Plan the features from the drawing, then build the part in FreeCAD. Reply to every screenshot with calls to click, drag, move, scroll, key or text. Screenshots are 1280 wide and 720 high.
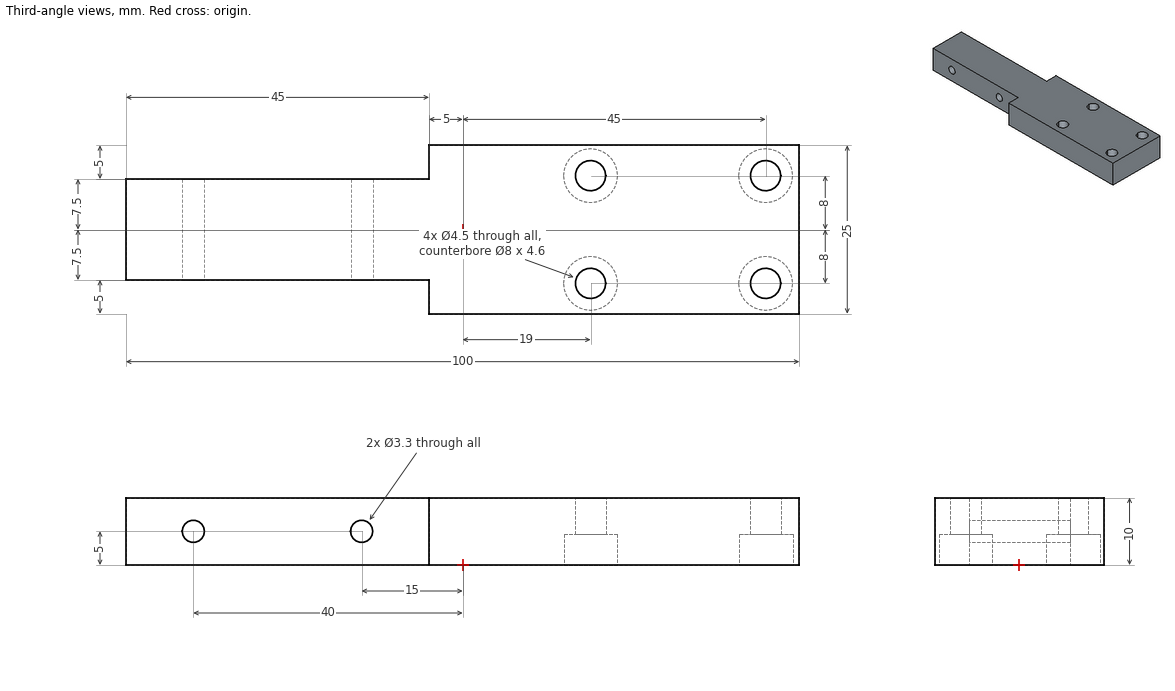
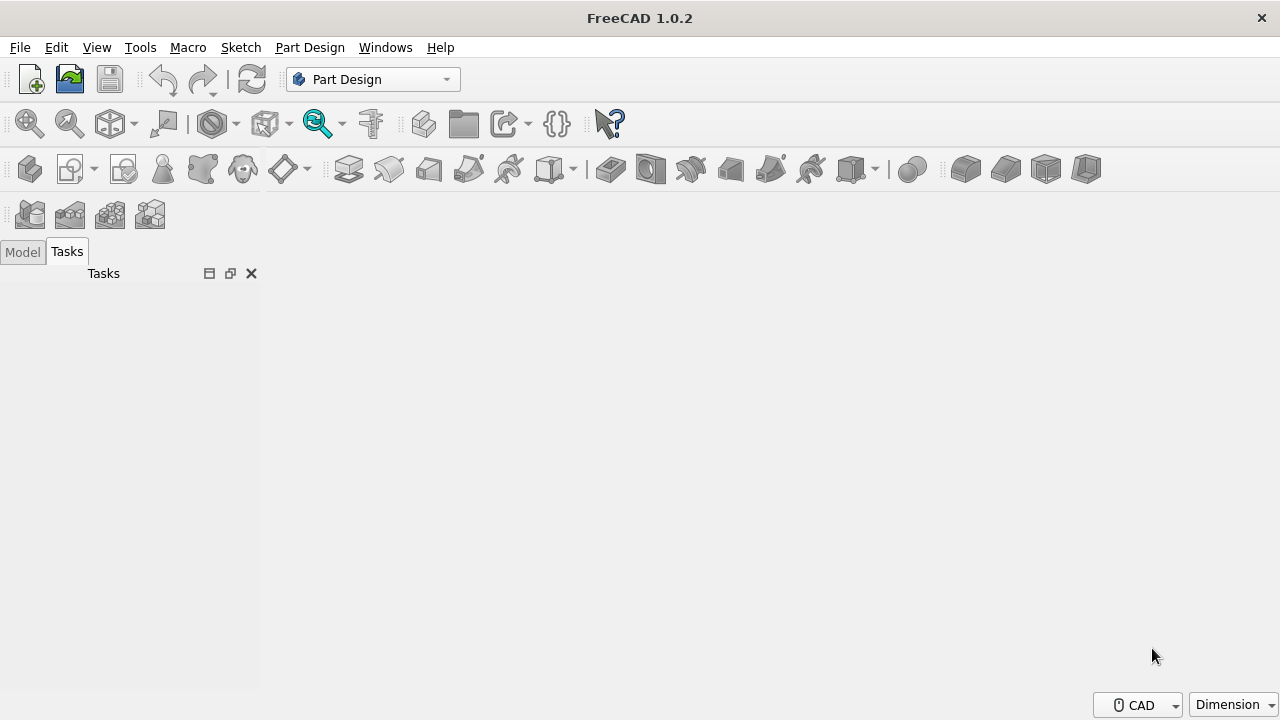
click(548, 80)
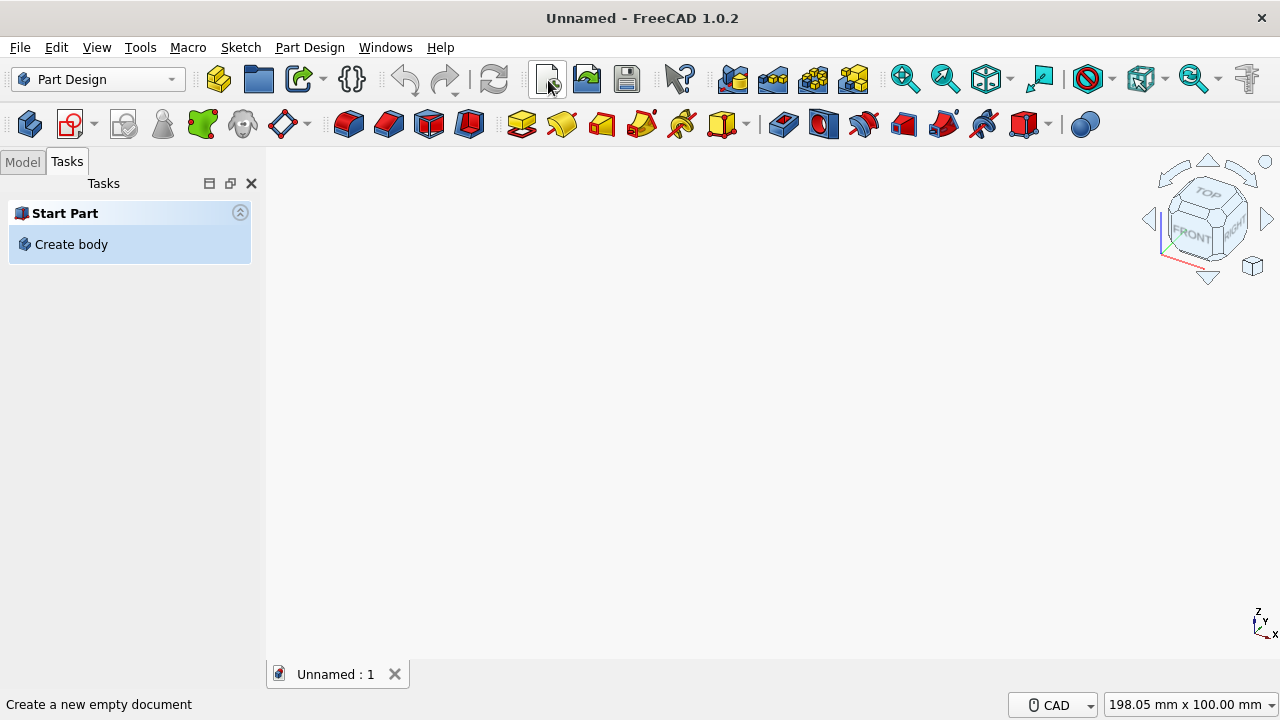
click(70, 124)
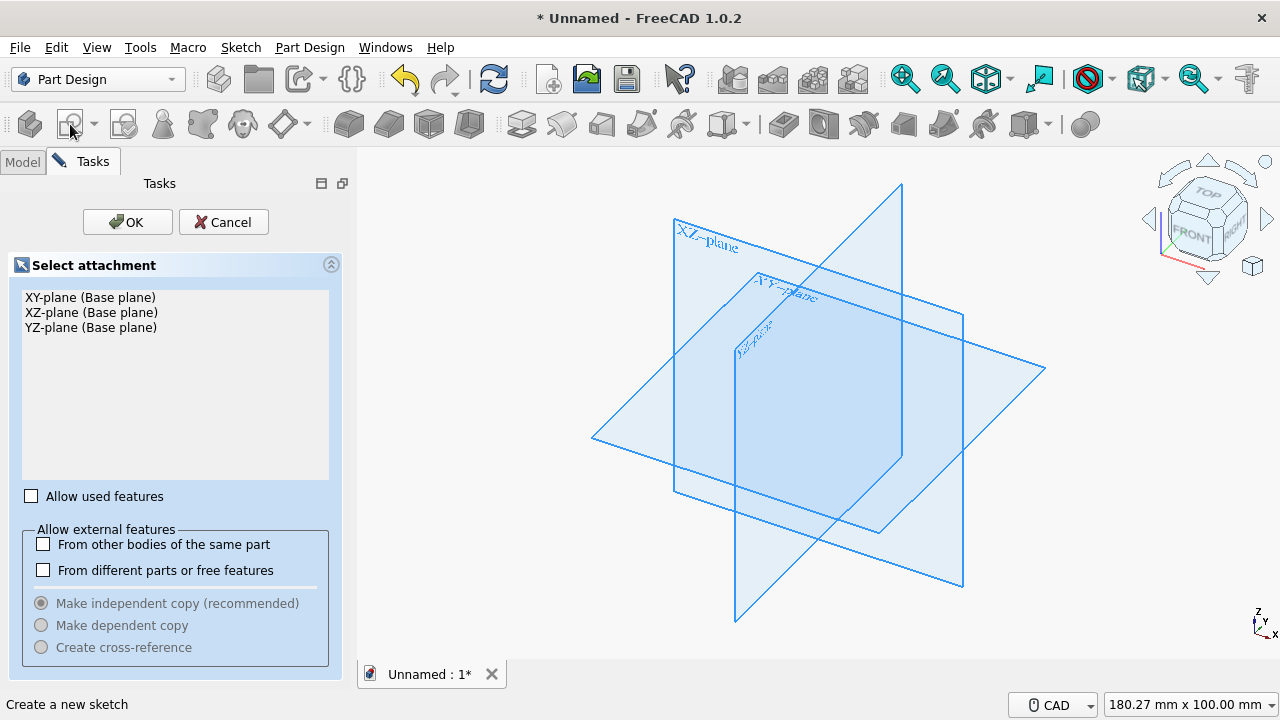
click(82, 298)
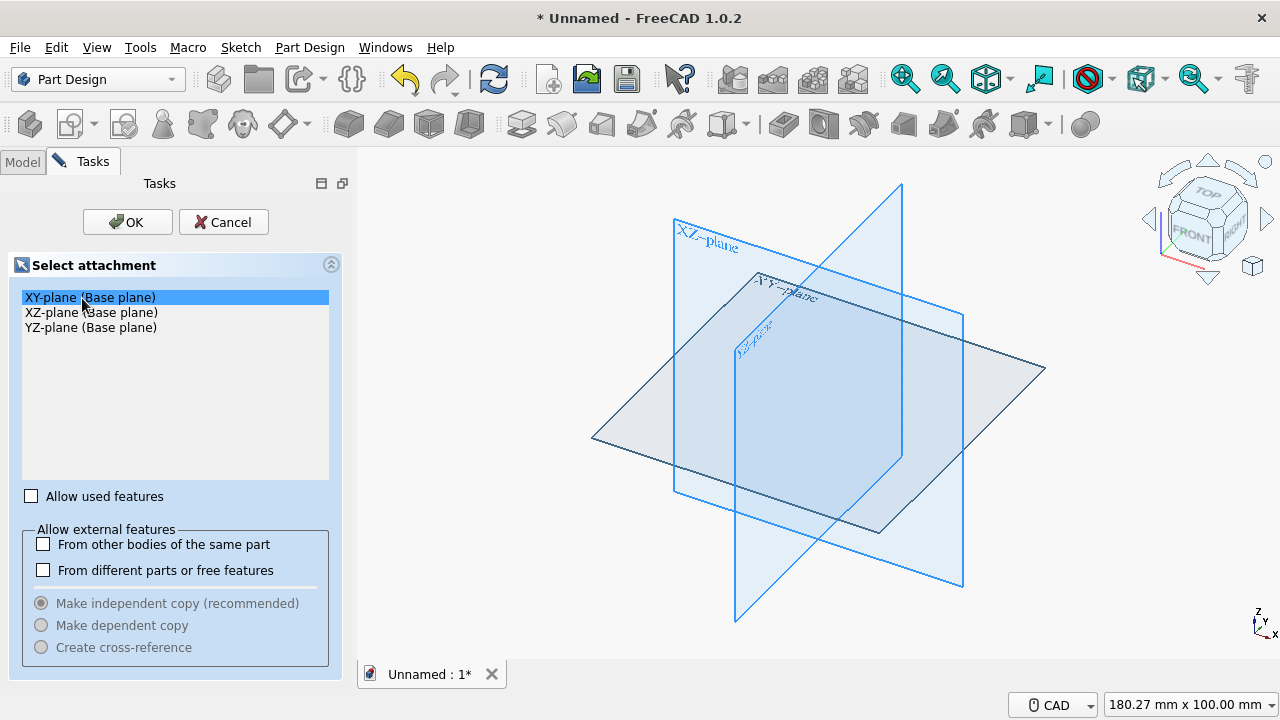
click(128, 222)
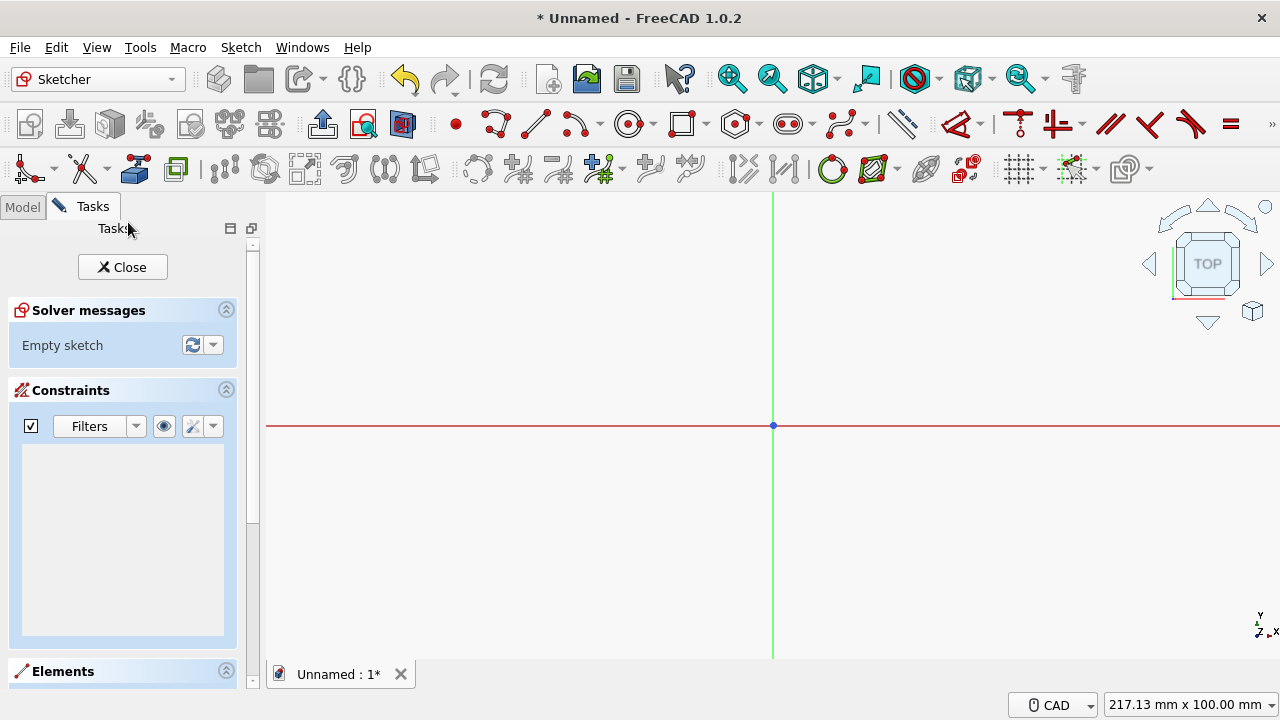
click(708, 124)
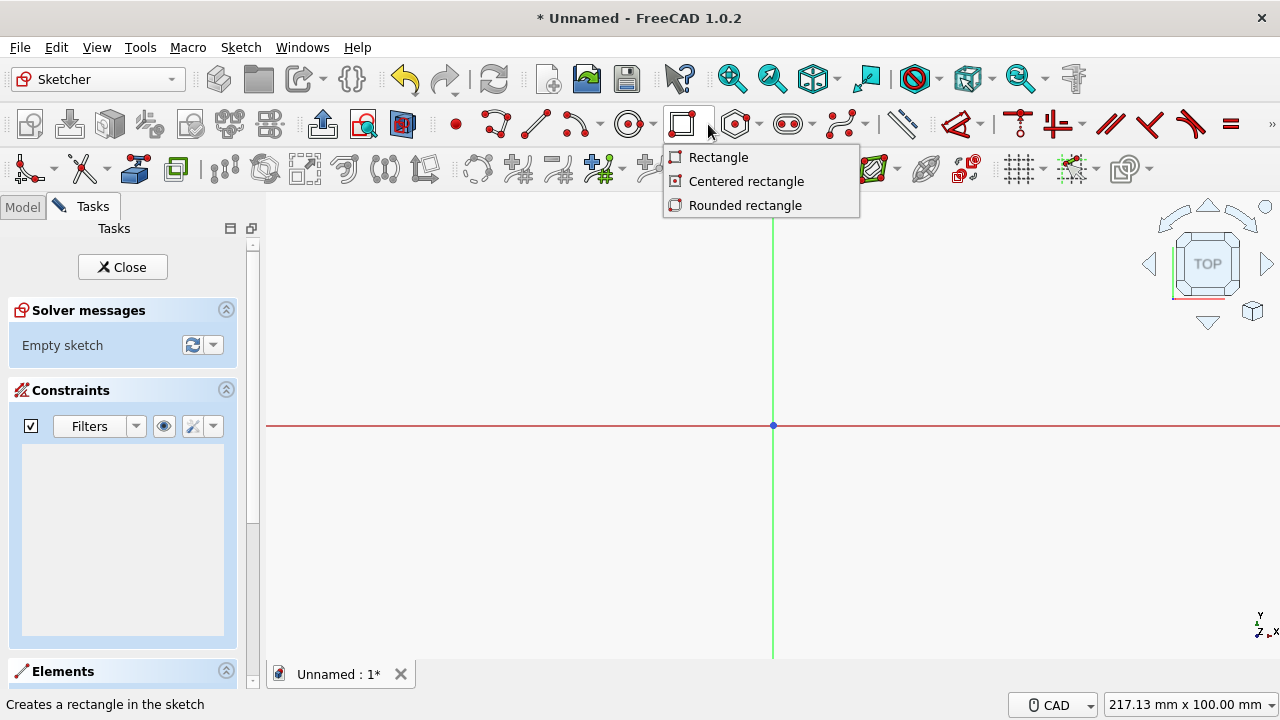
click(762, 181)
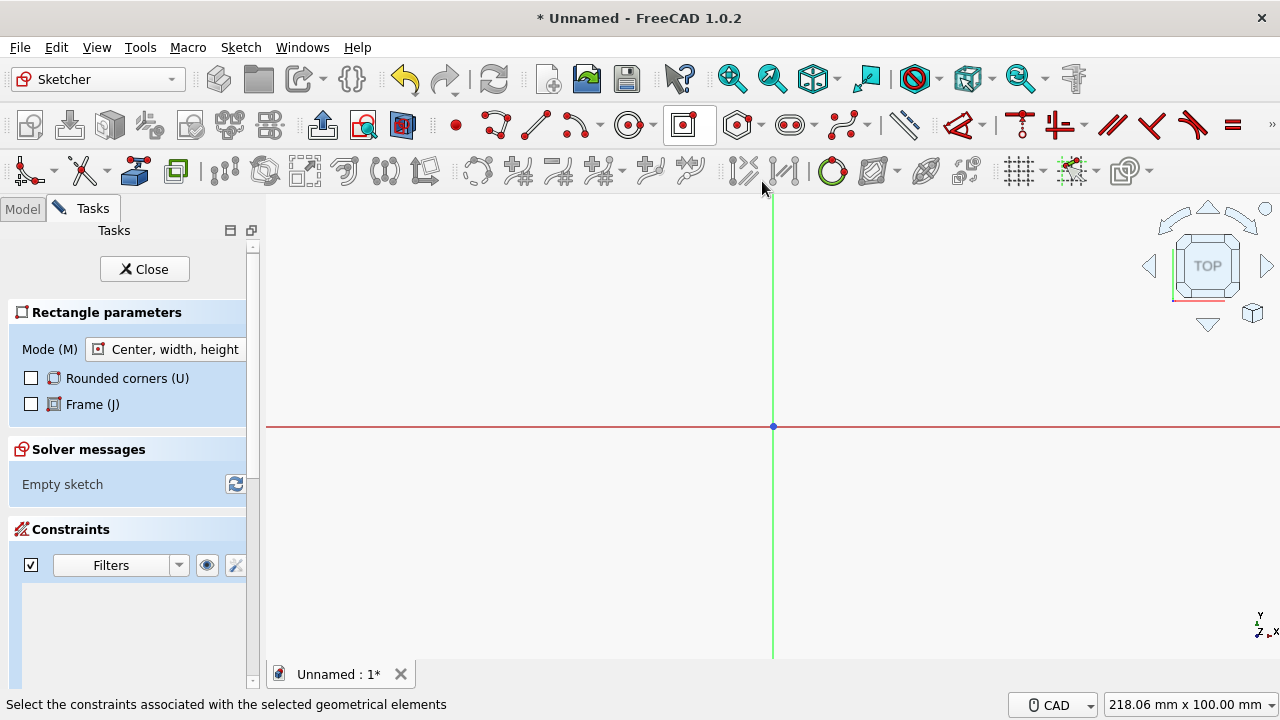
click(773, 426)
click(1006, 368)
key(Escape)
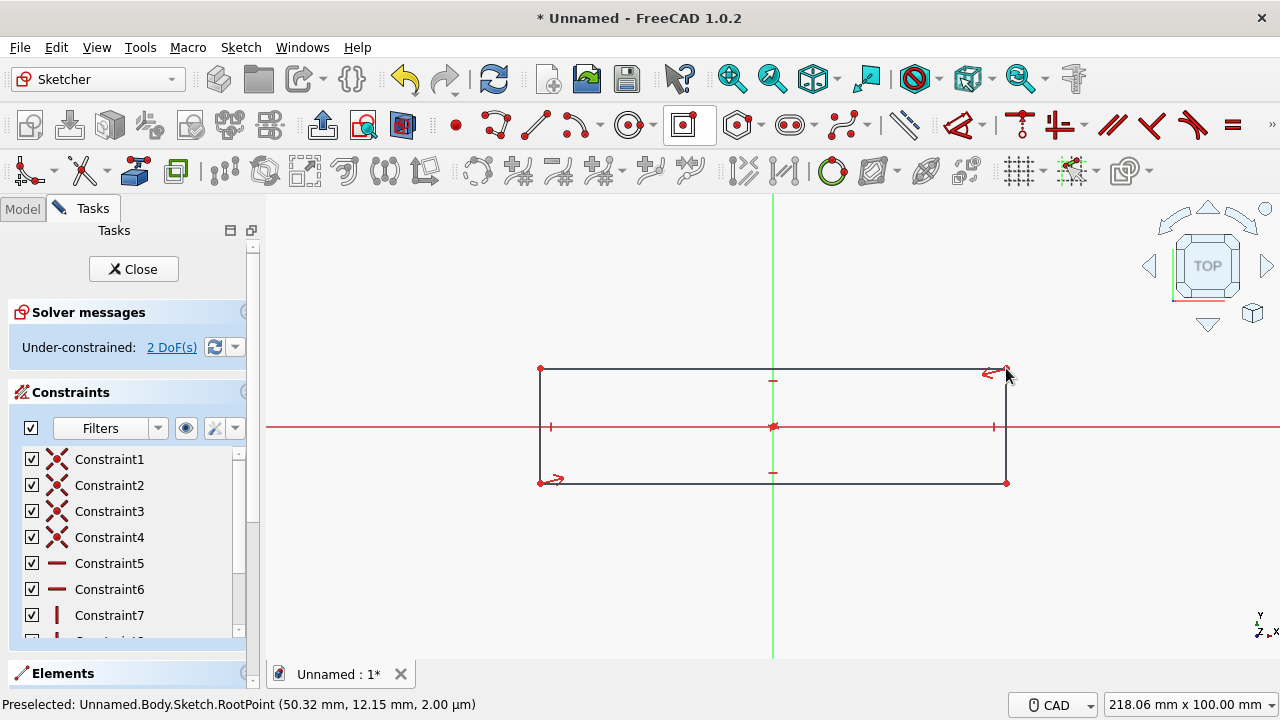
click(958, 126)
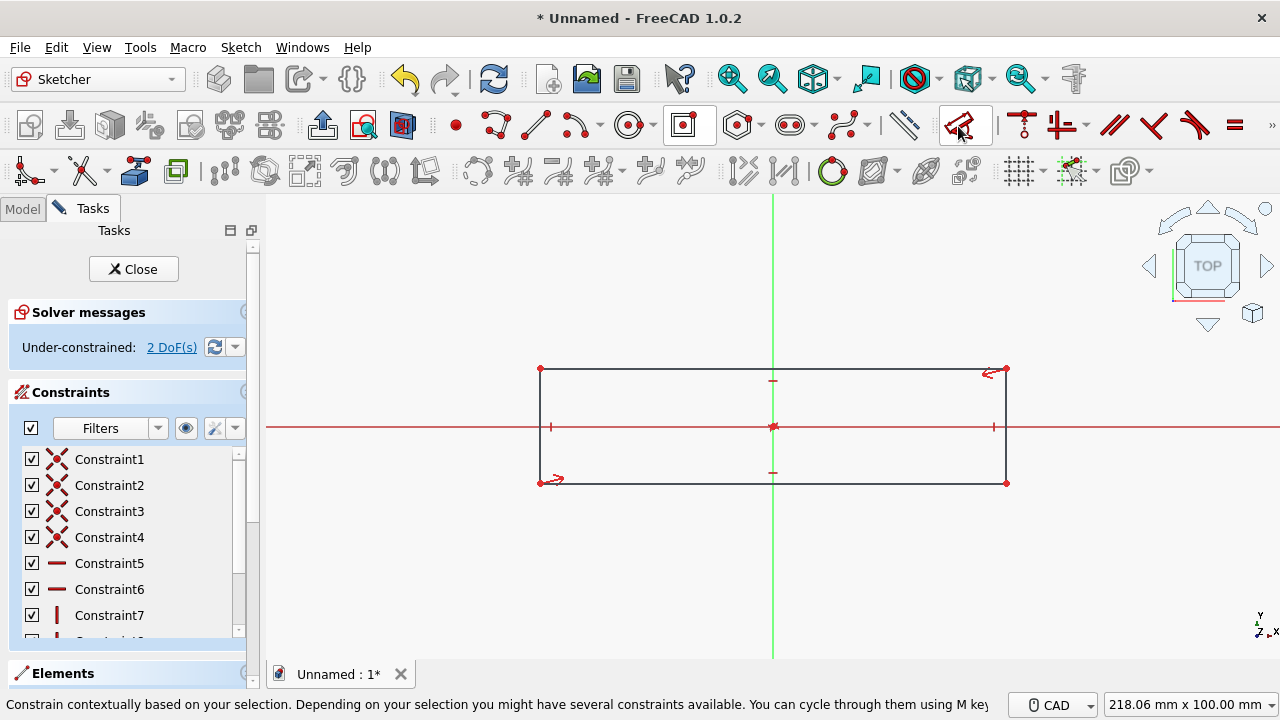
click(1006, 449)
click(1040, 400)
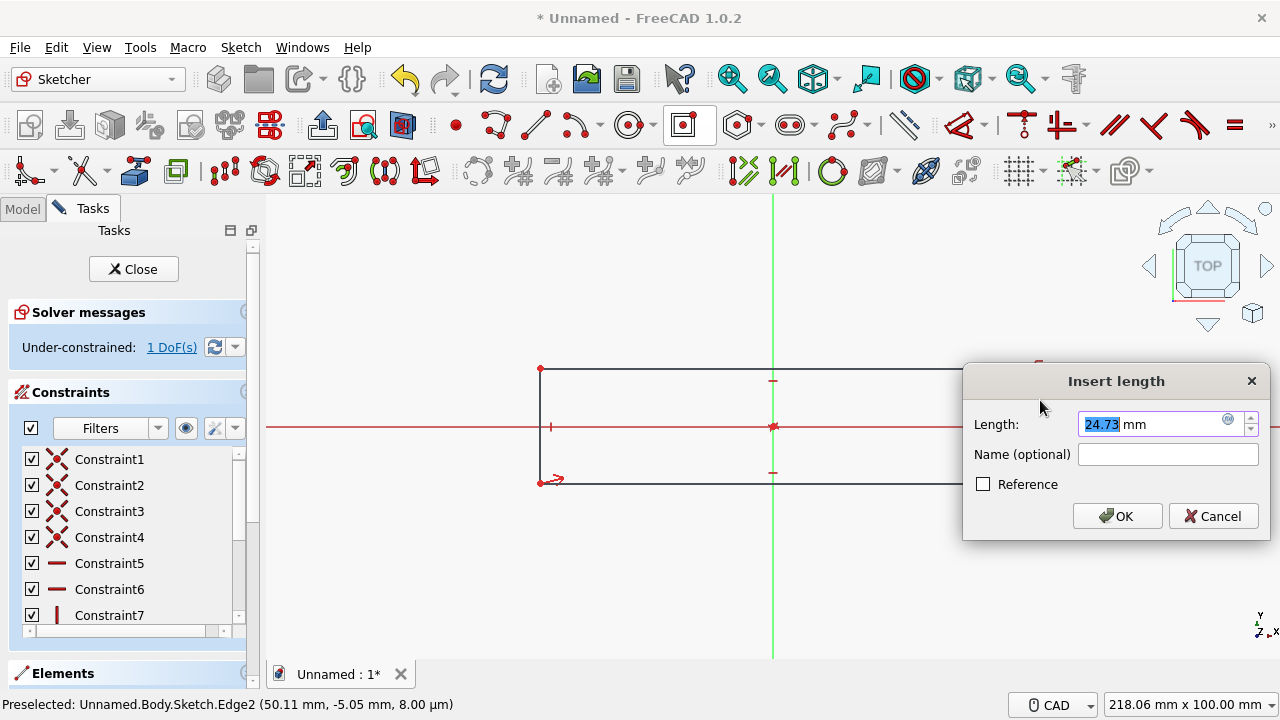
text(25)
key(Return)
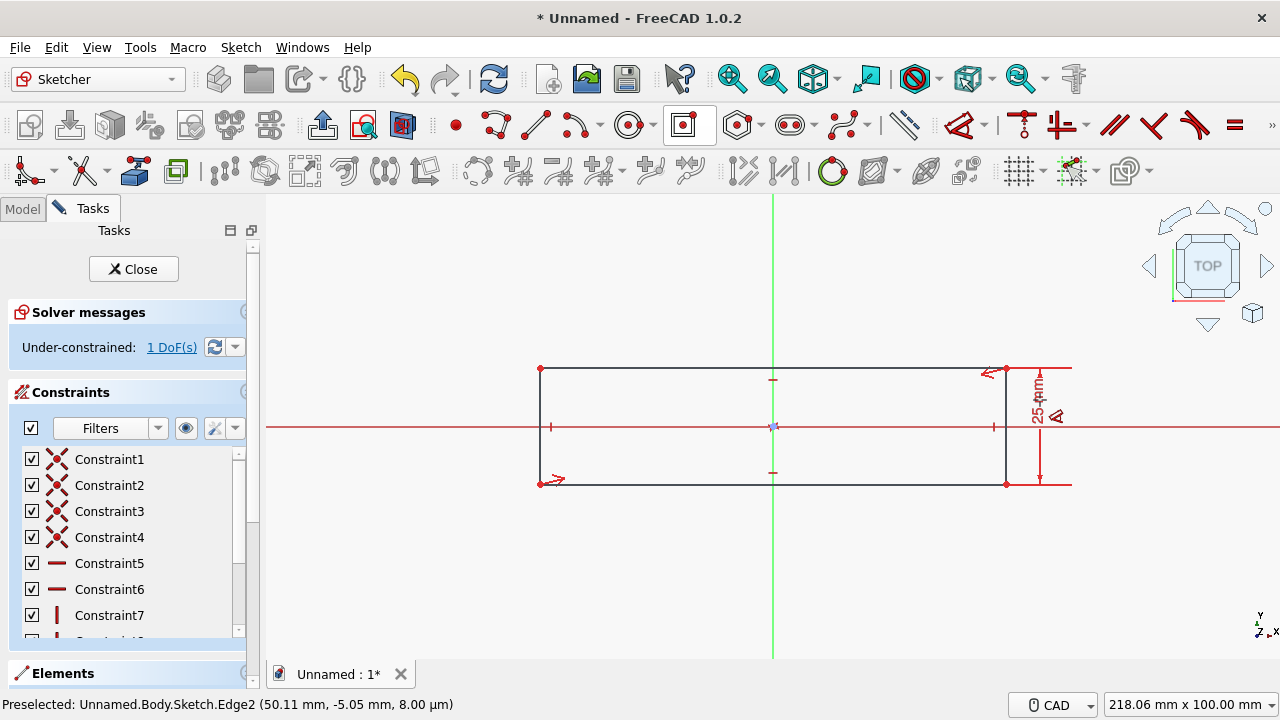
click(680, 485)
click(666, 519)